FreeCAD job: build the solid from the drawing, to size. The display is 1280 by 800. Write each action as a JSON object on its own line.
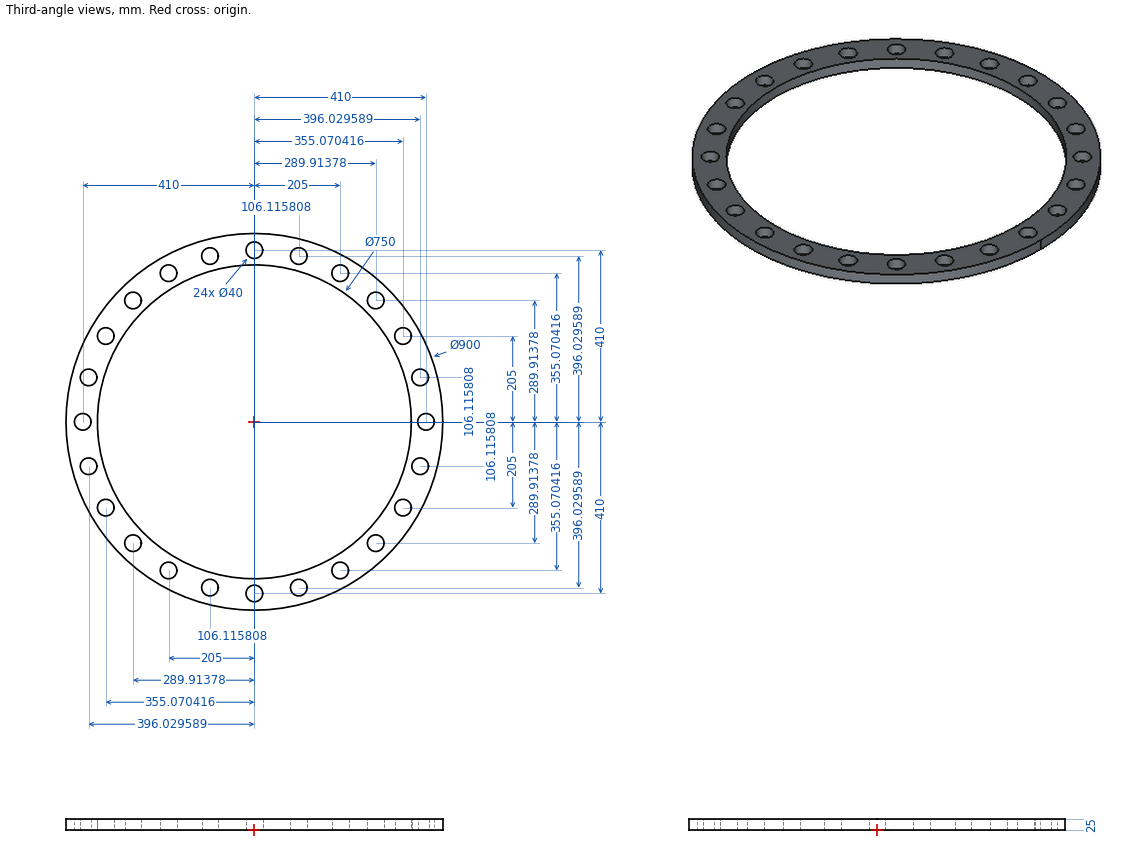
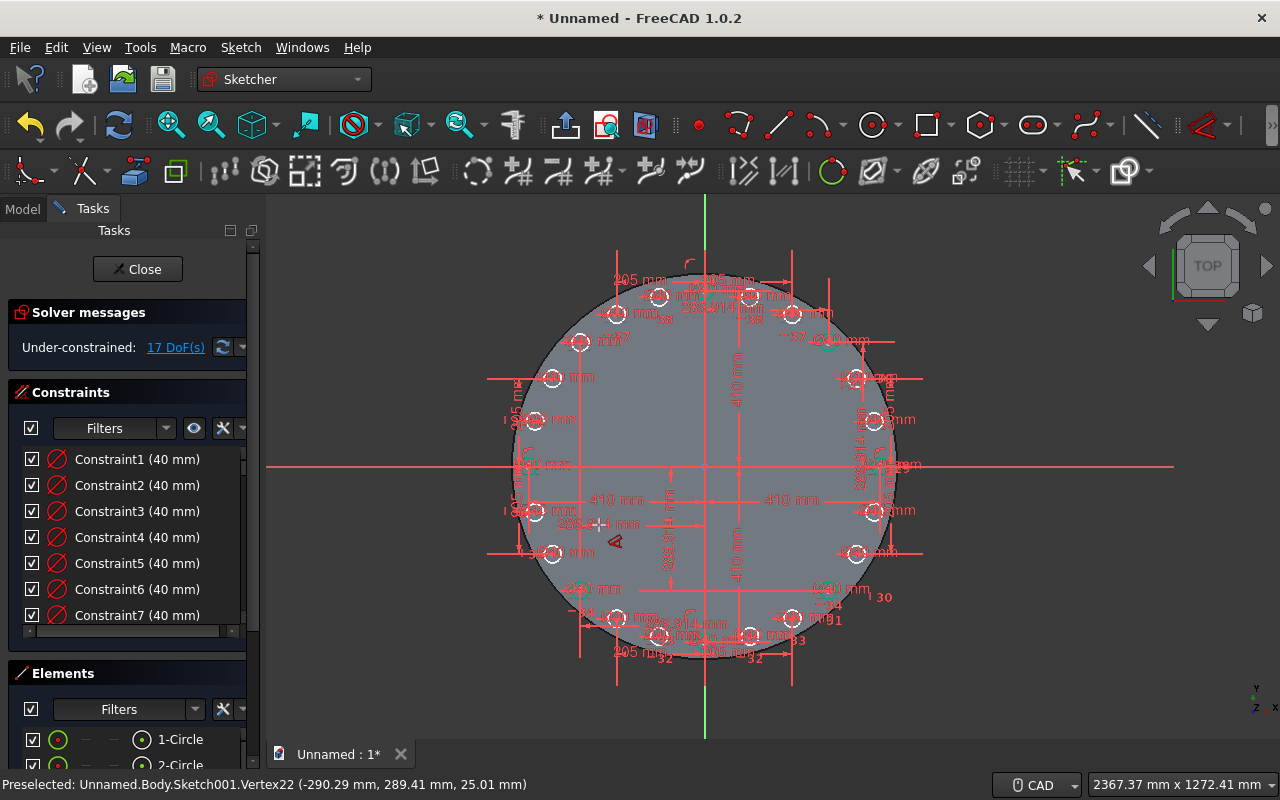
{"action": "left_click", "coordinate": [580, 343]}
{"action": "left_click", "coordinate": [546, 448]}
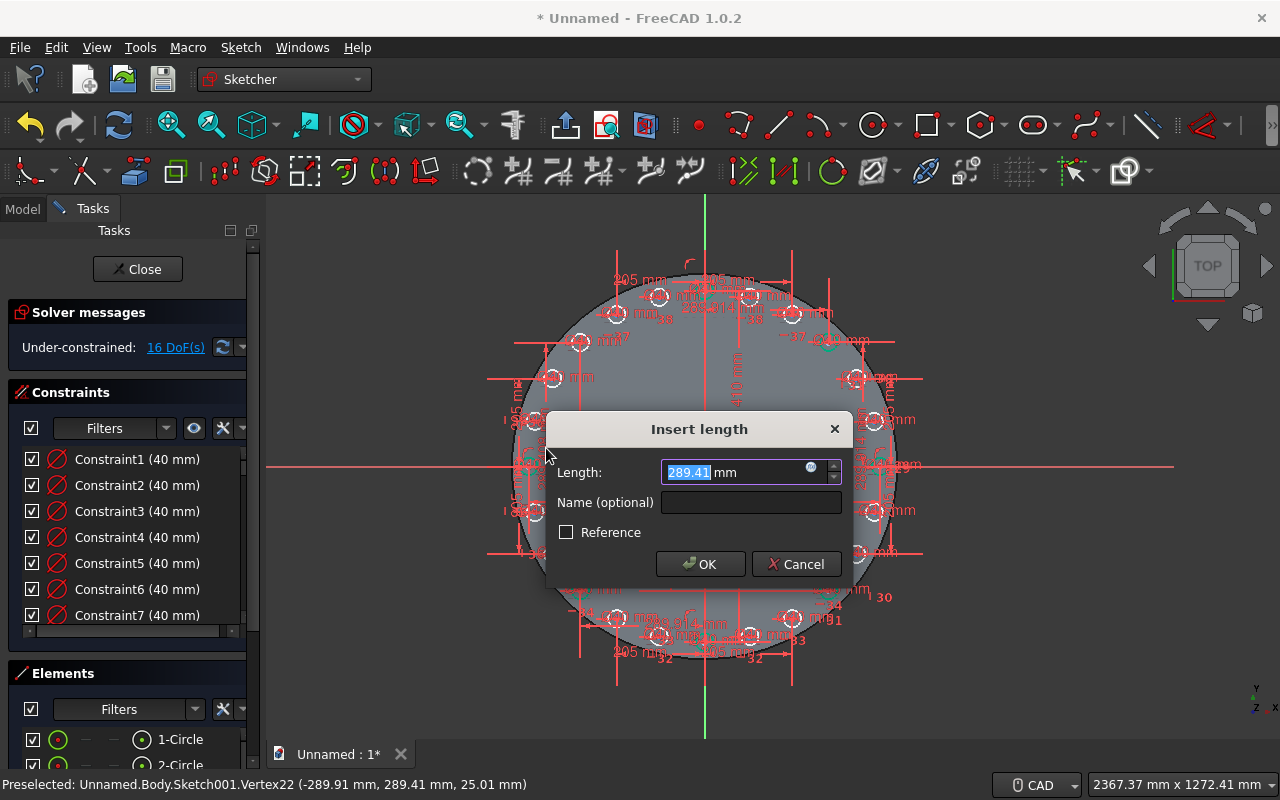
{"action": "type", "text": "289.91378"}
{"action": "key", "text": "Return"}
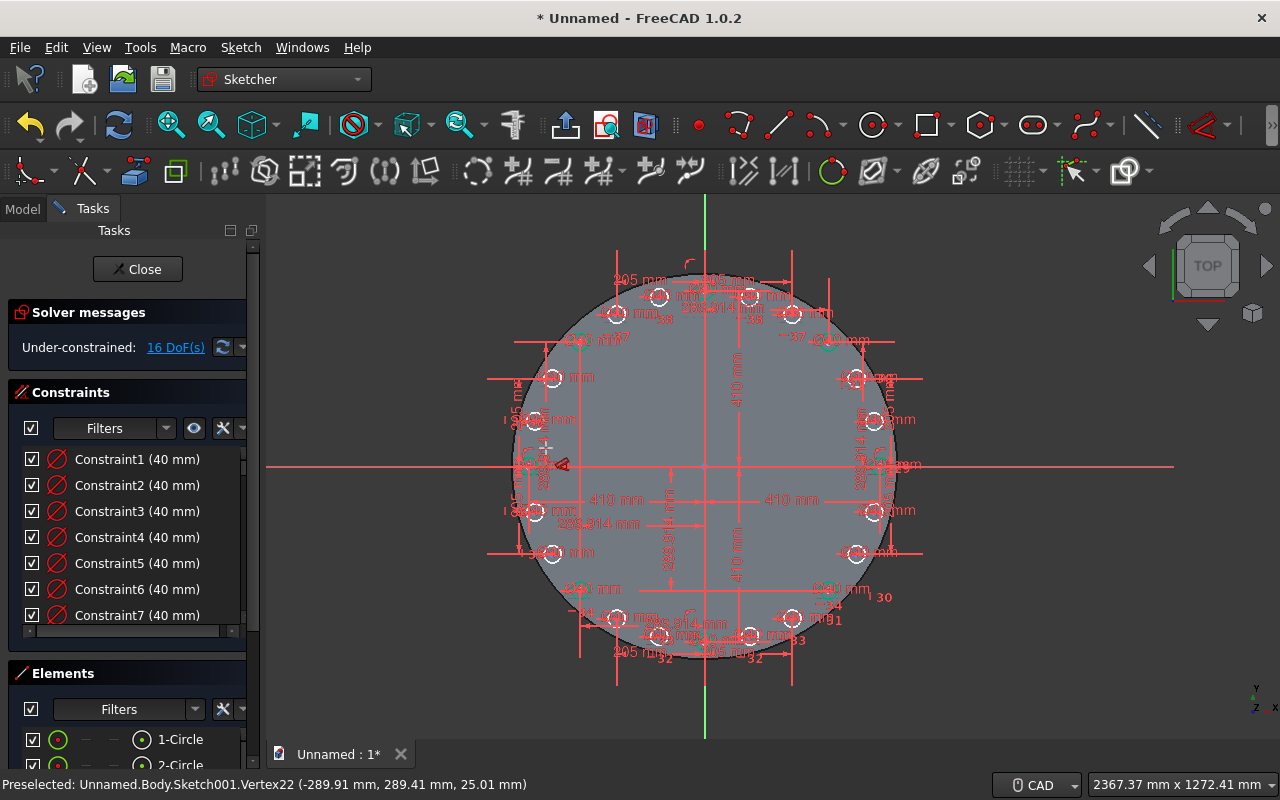
{"action": "left_click", "coordinate": [750, 297]}
{"action": "left_click", "coordinate": [727, 239]}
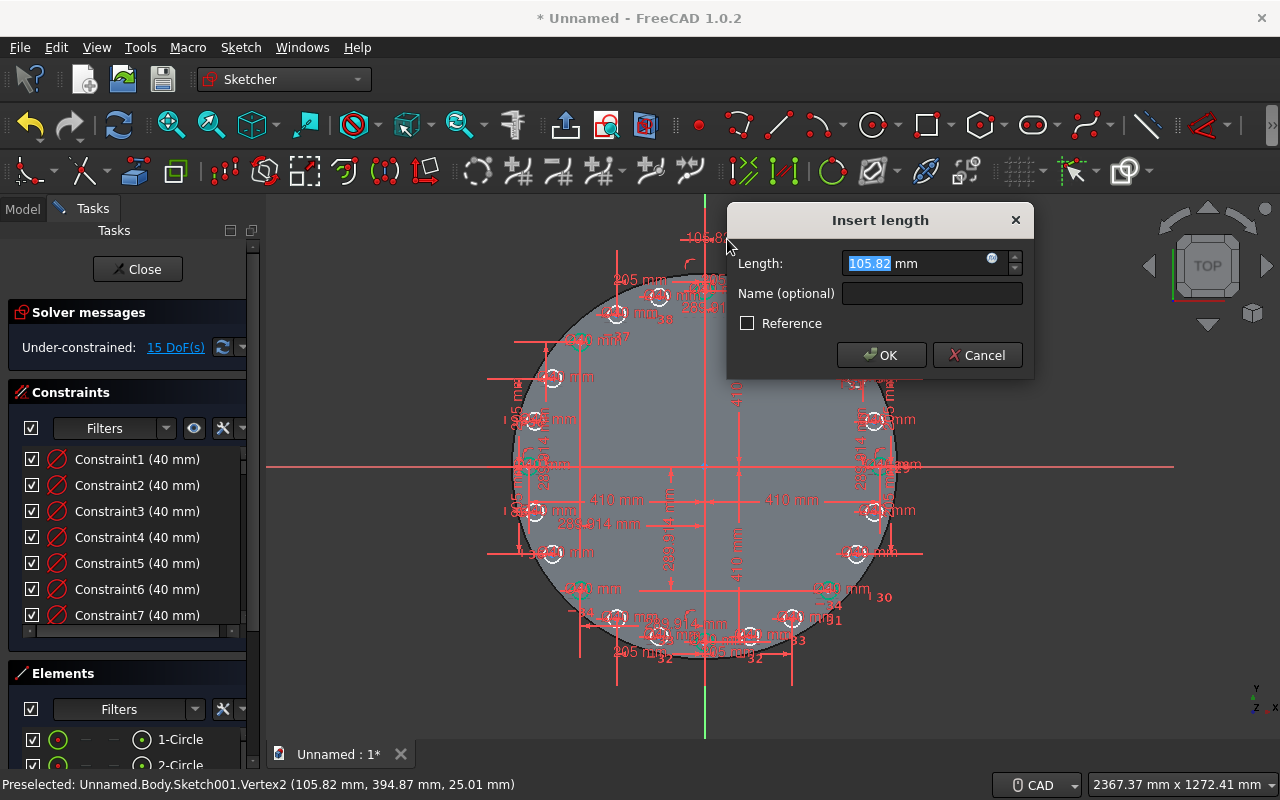
{"action": "type", "text": "106.115808"}
{"action": "key", "text": "Return"}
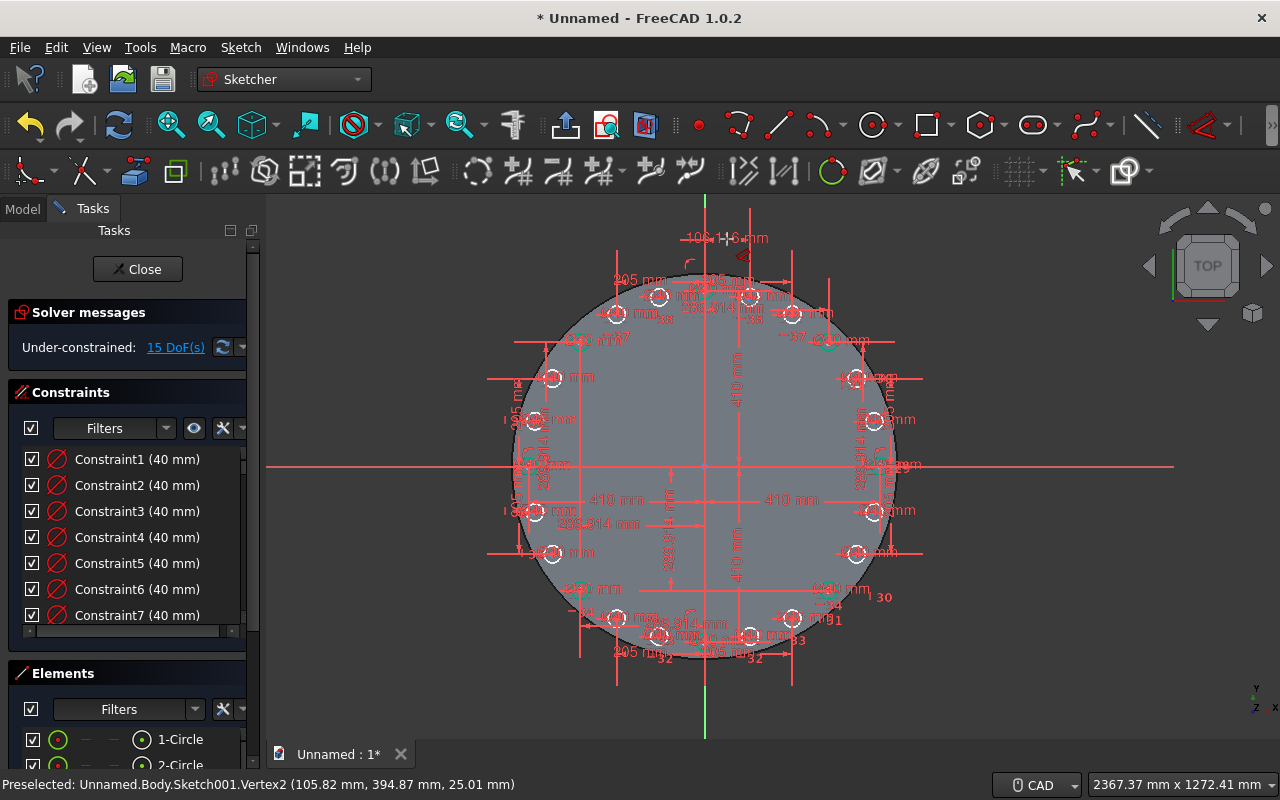
{"action": "left_click", "coordinate": [750, 297]}
{"action": "left_click", "coordinate": [784, 343]}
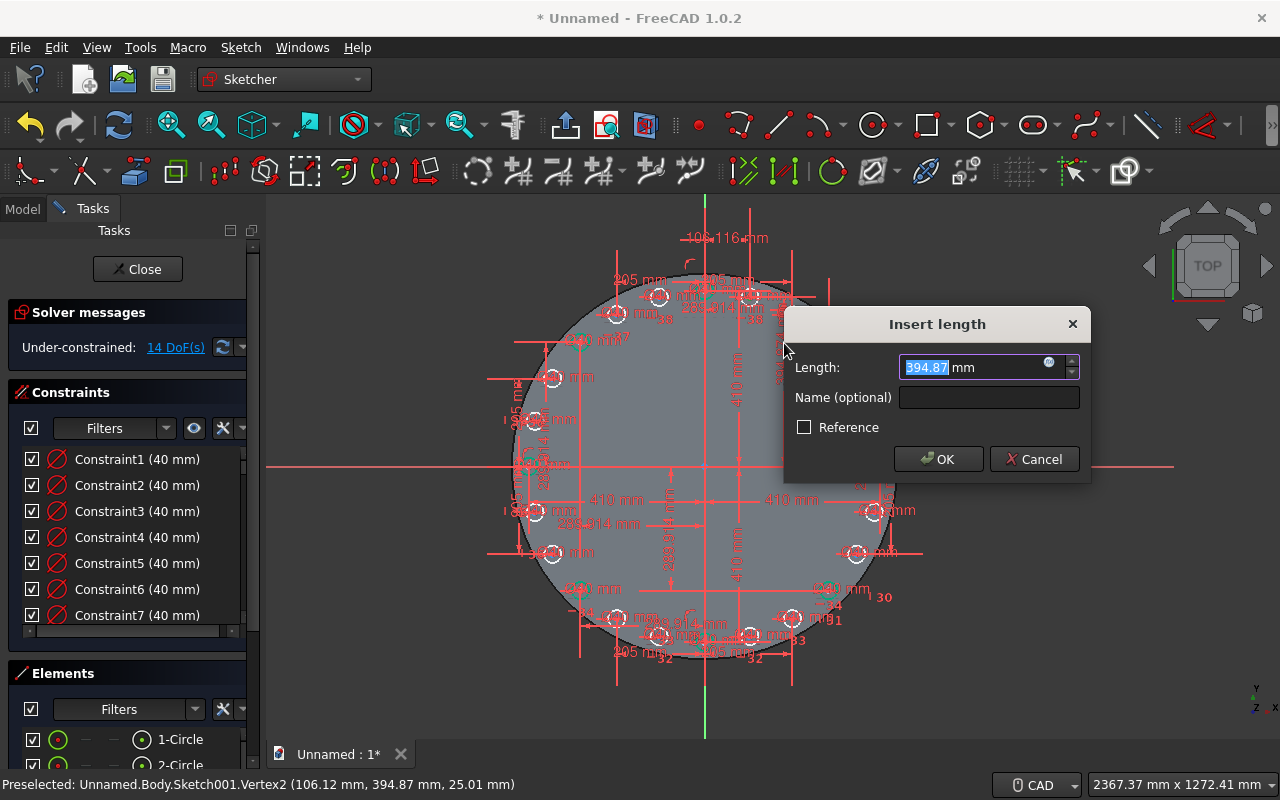
{"action": "type", "text": "396.029589"}
{"action": "key", "text": "Return"}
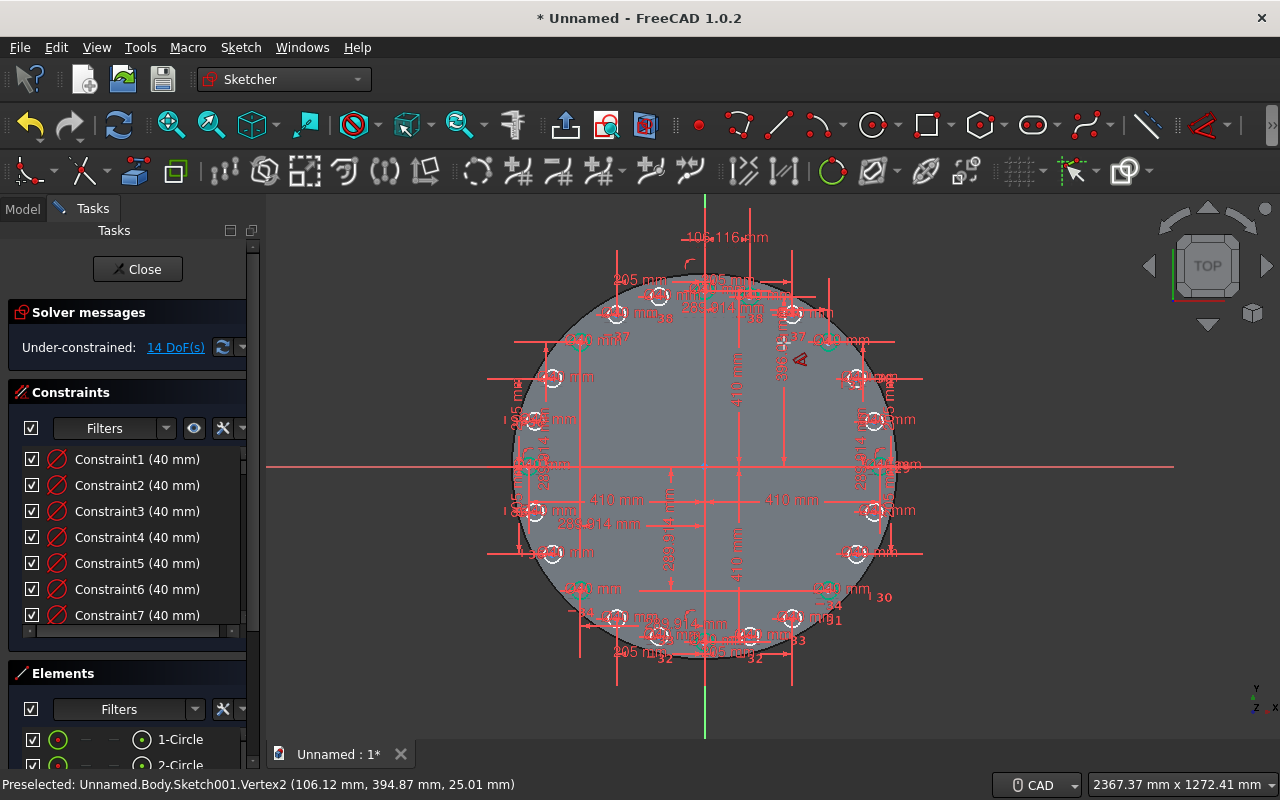
{"action": "left_click", "coordinate": [792, 315]}
{"action": "left_click", "coordinate": [826, 426]}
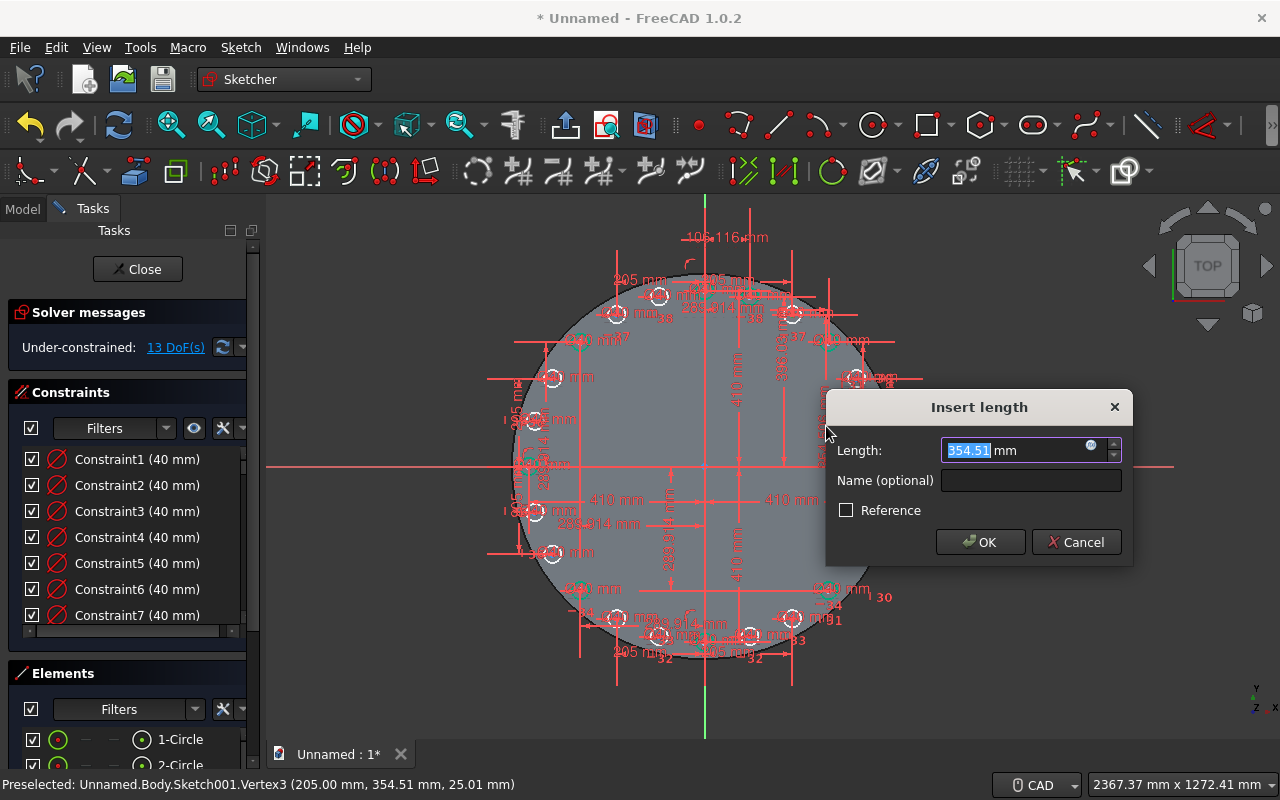
{"action": "type", "text": "355.070416"}
{"action": "key", "text": "Return"}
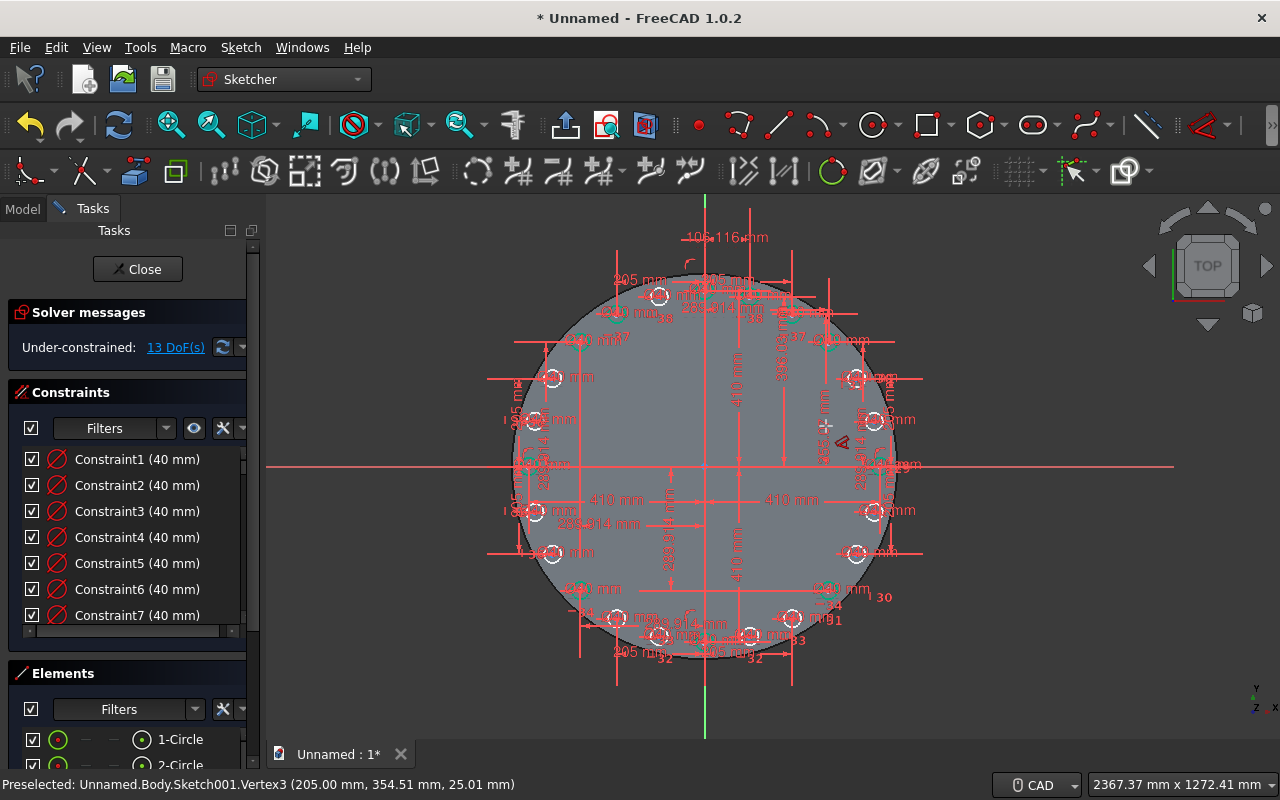
{"action": "left_click", "coordinate": [857, 379]}
{"action": "left_click", "coordinate": [816, 321]}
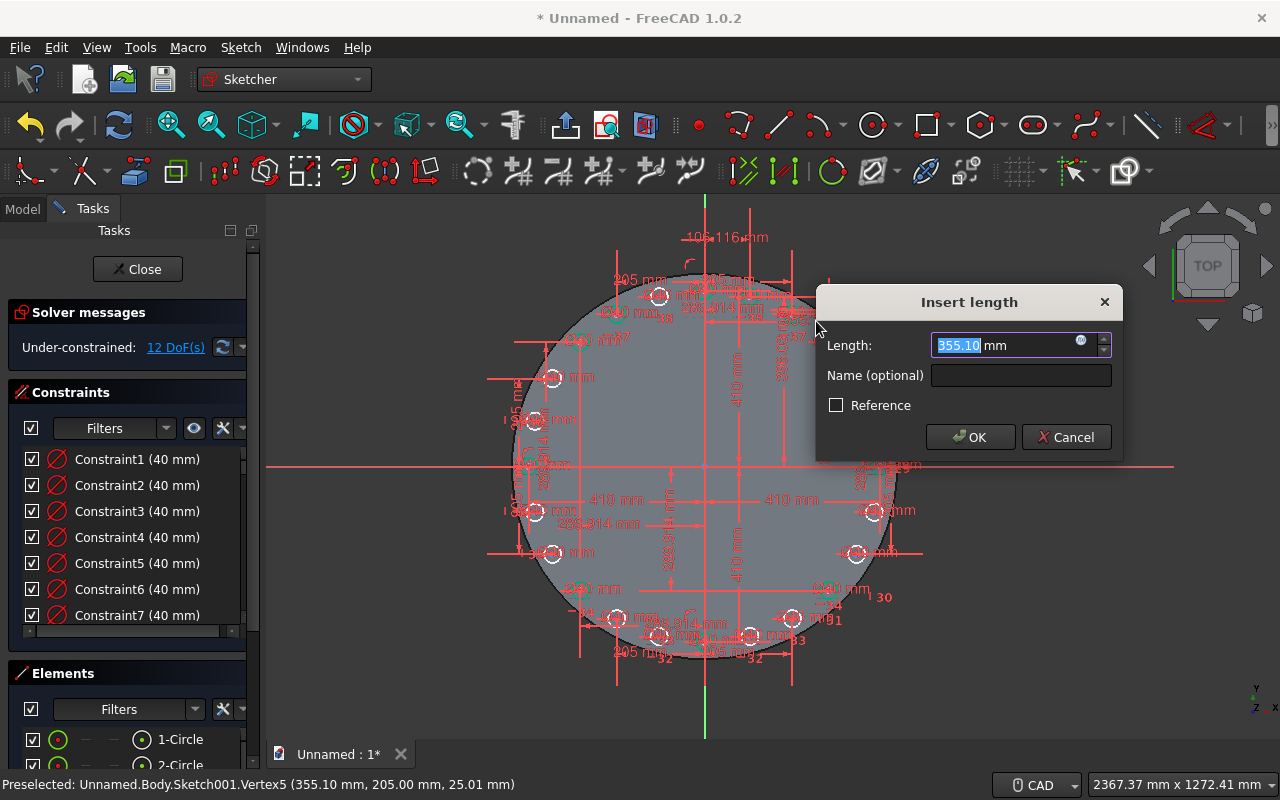
{"action": "type", "text": "355.070416"}
{"action": "key", "text": "Return"}